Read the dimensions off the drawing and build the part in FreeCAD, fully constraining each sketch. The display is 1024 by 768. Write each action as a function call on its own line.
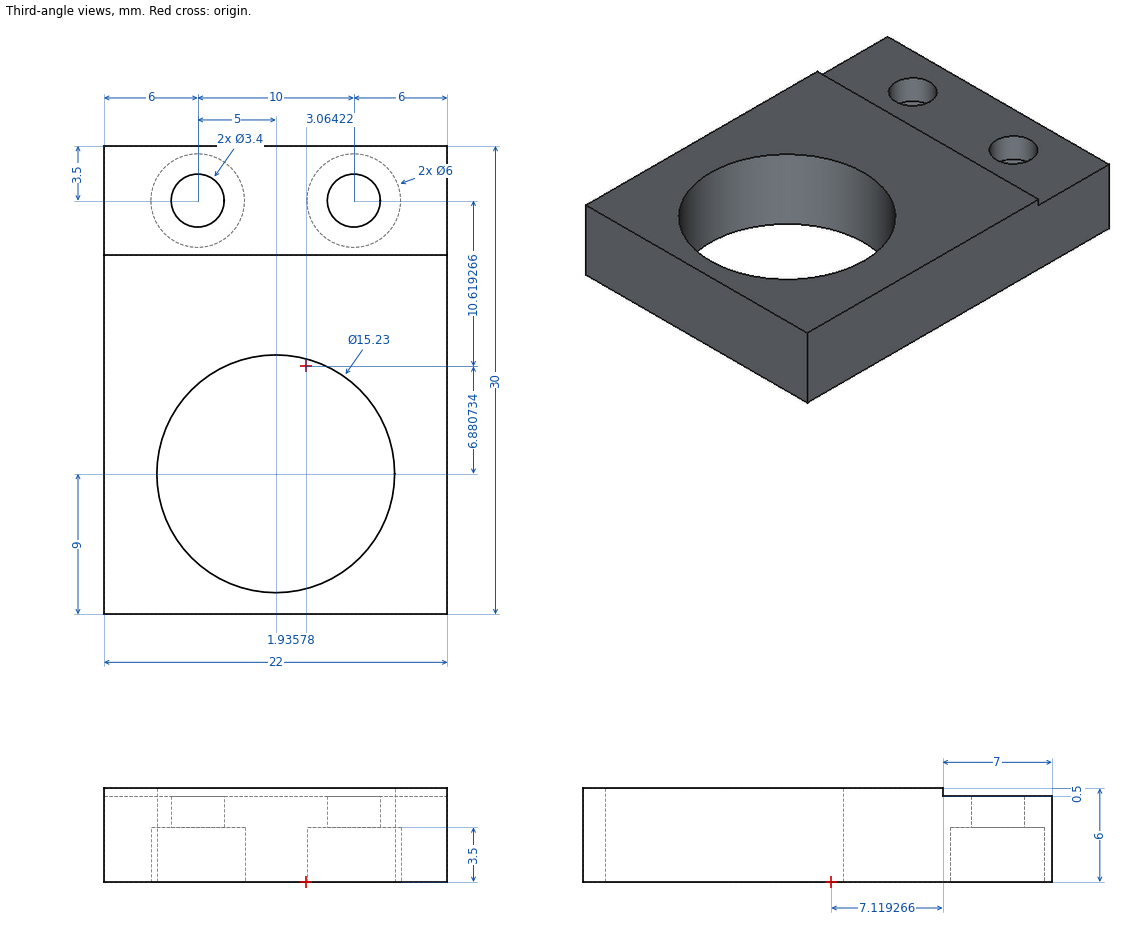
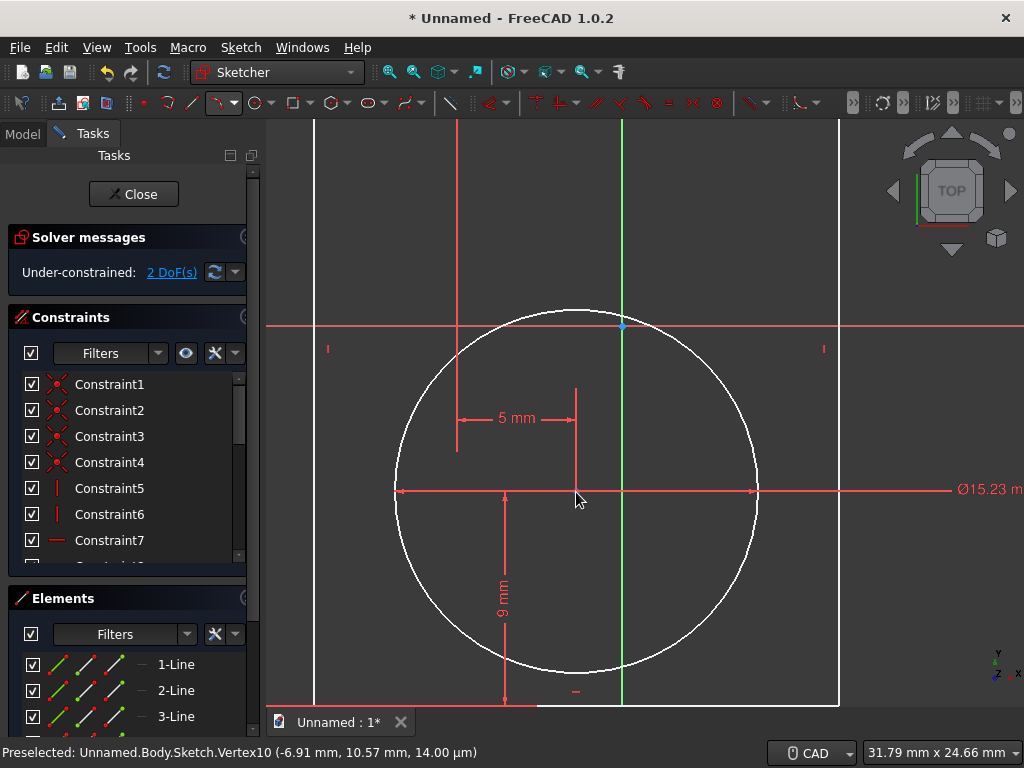
click(576, 491)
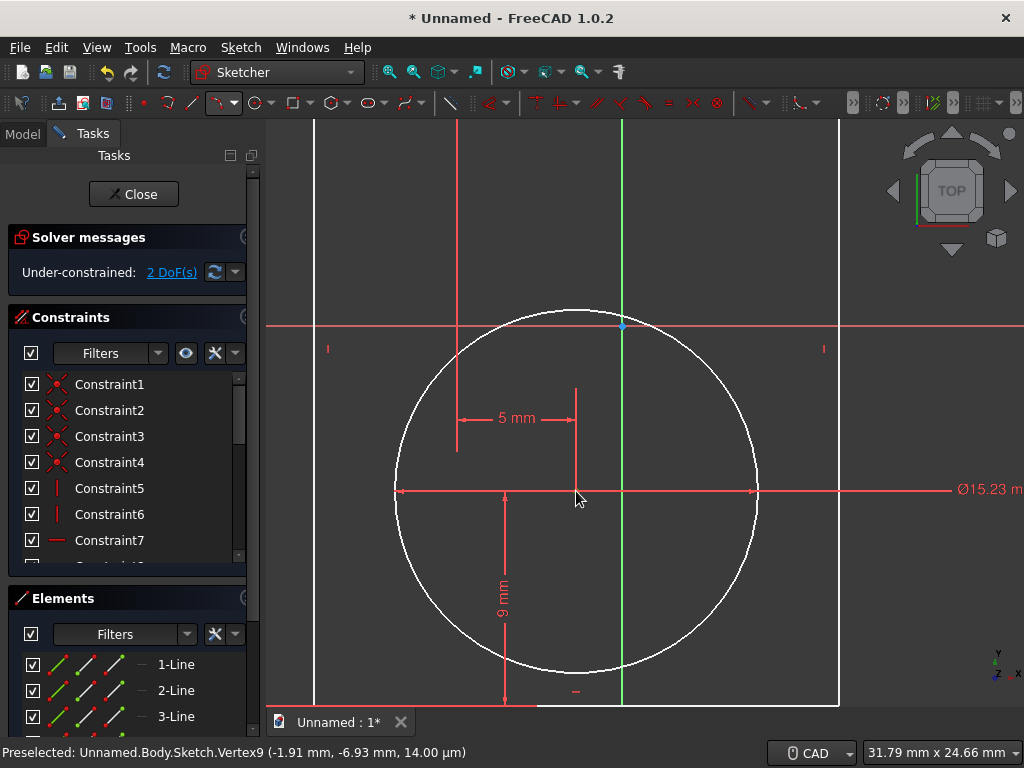
key(l)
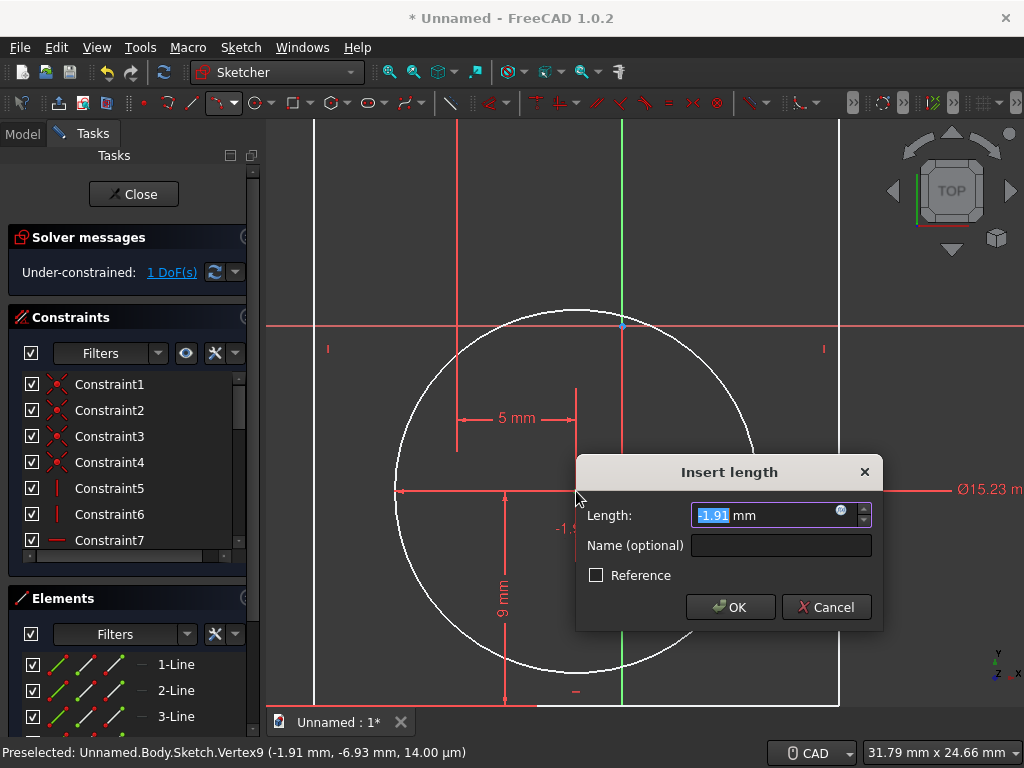
text(-1.93578)
key(Return)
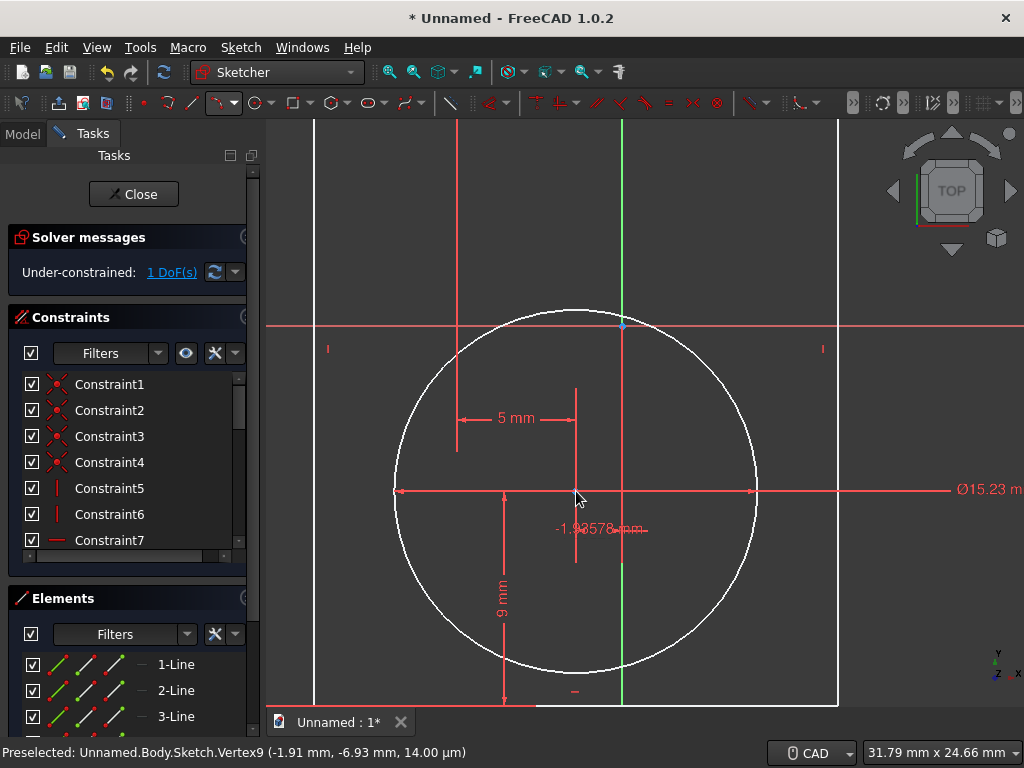
click(576, 491)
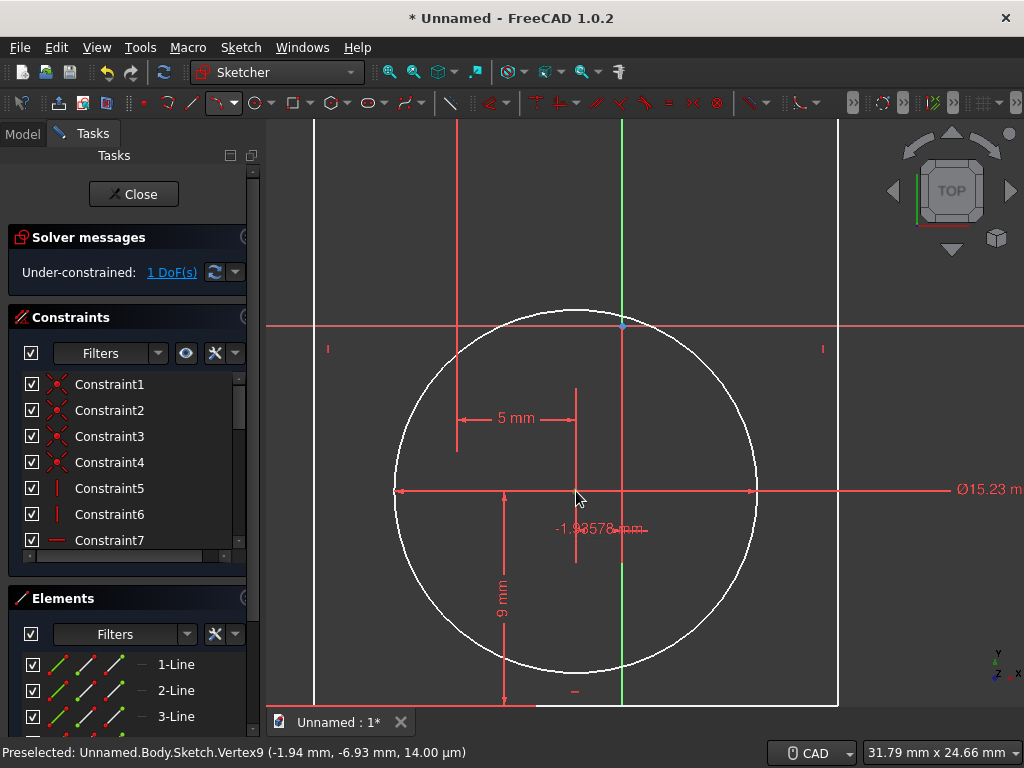
key(i)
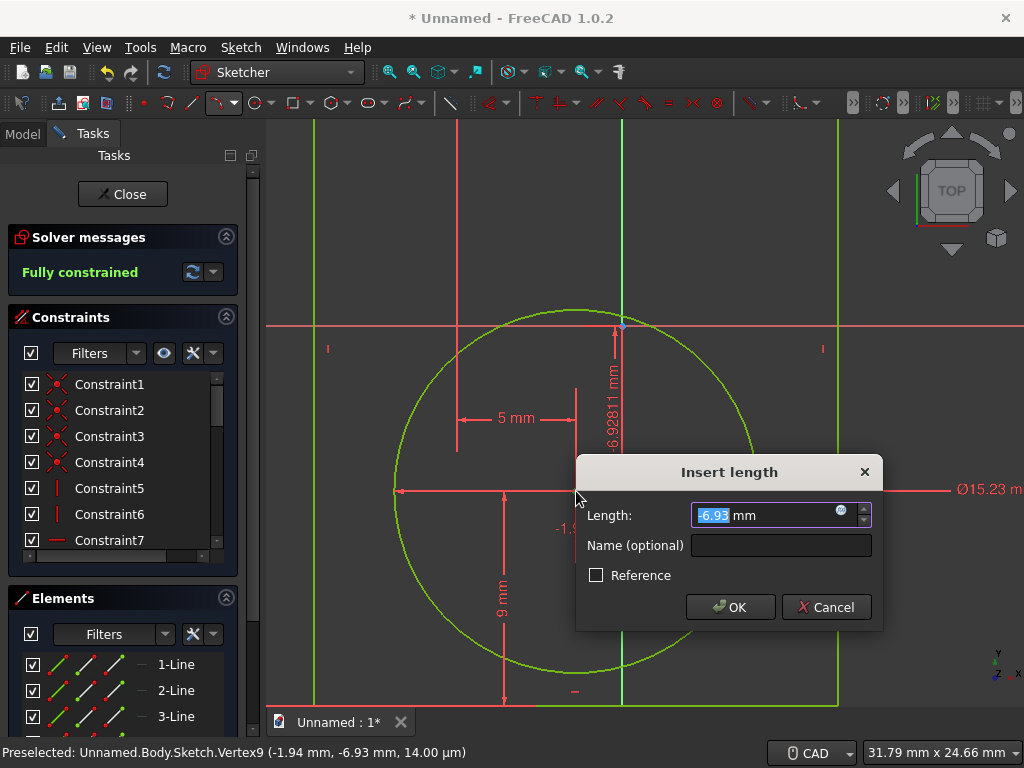
text(-6.880734)
key(Return)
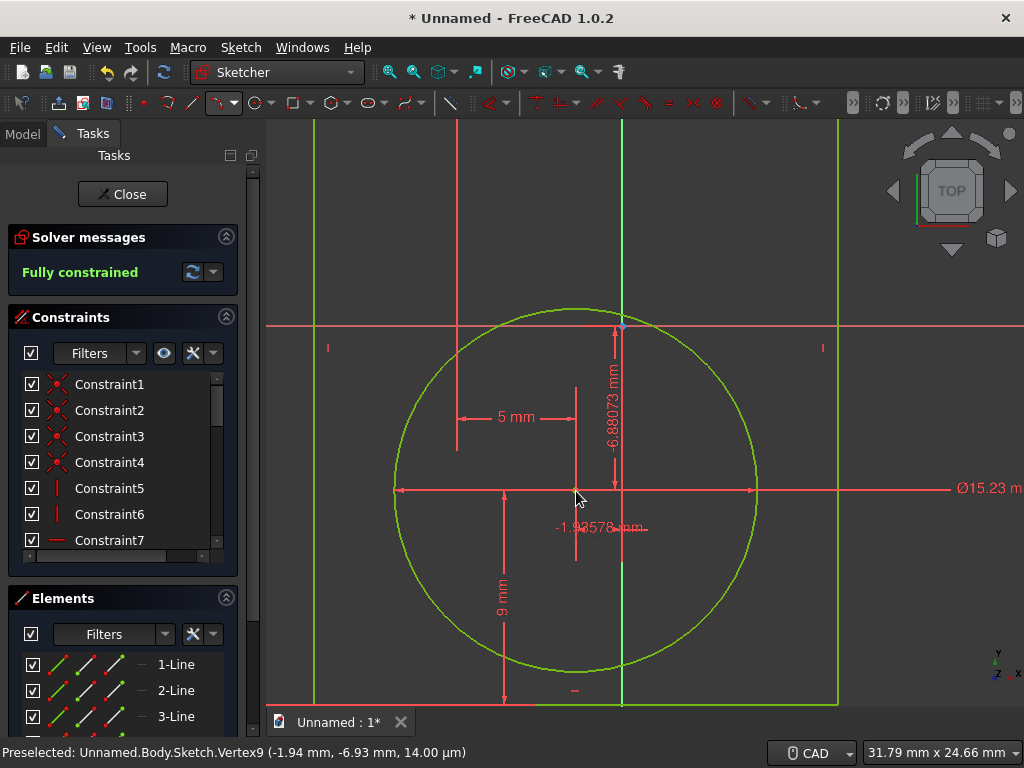
click(123, 194)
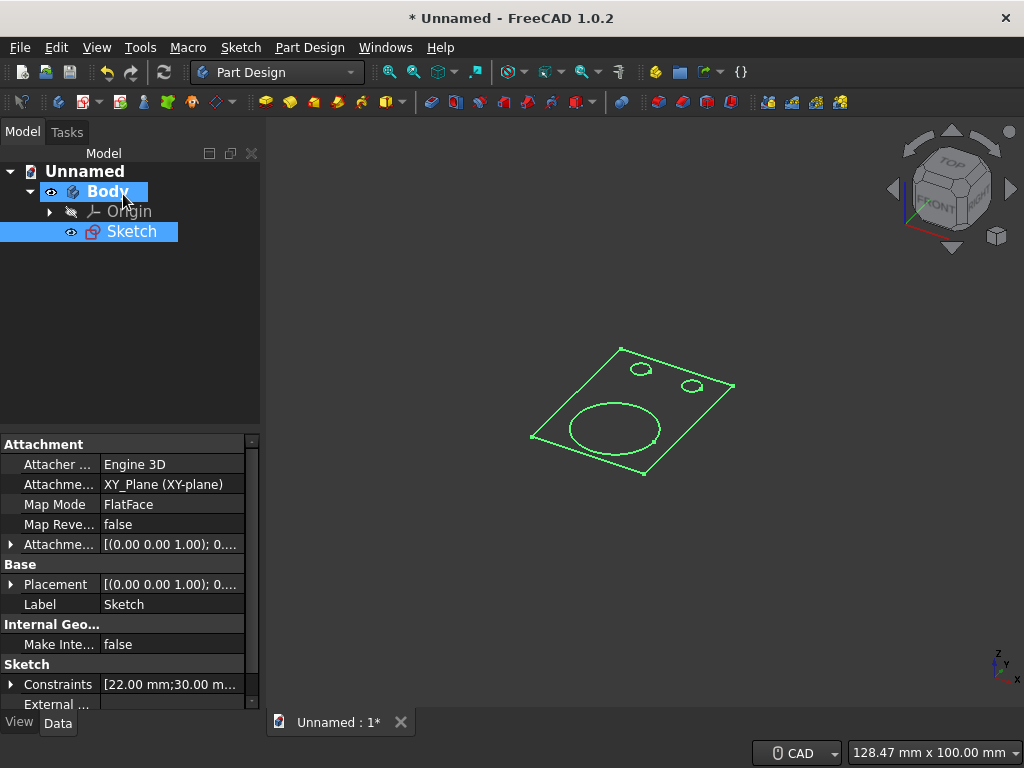
click(266, 102)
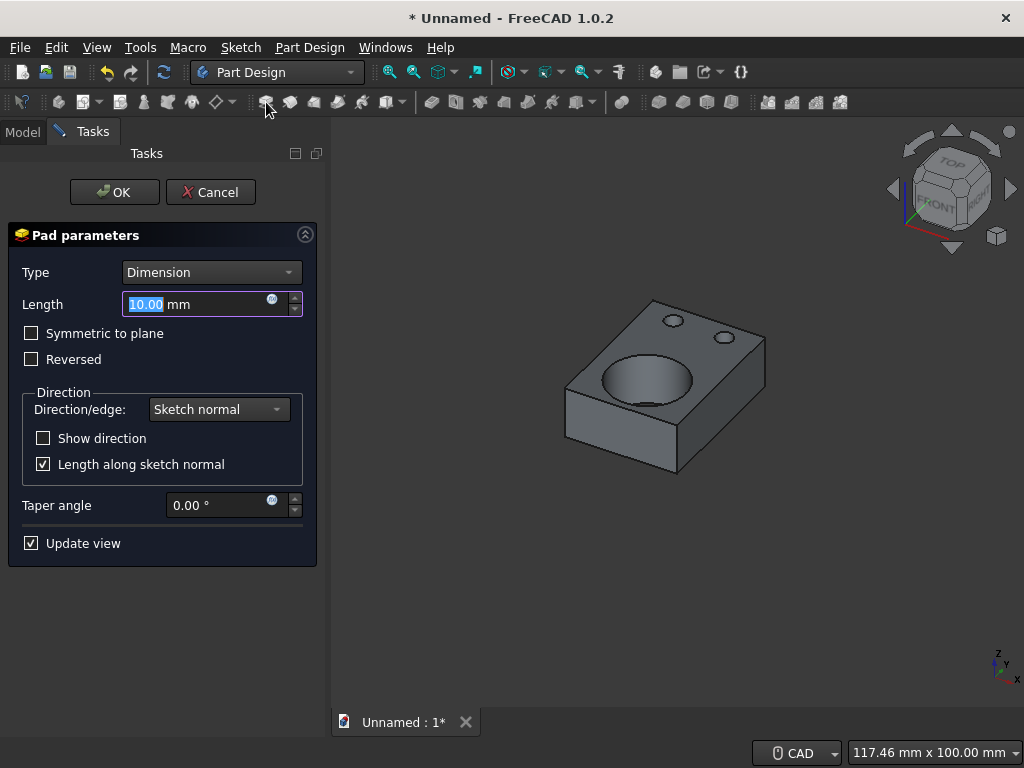
text(6)
key(Tab)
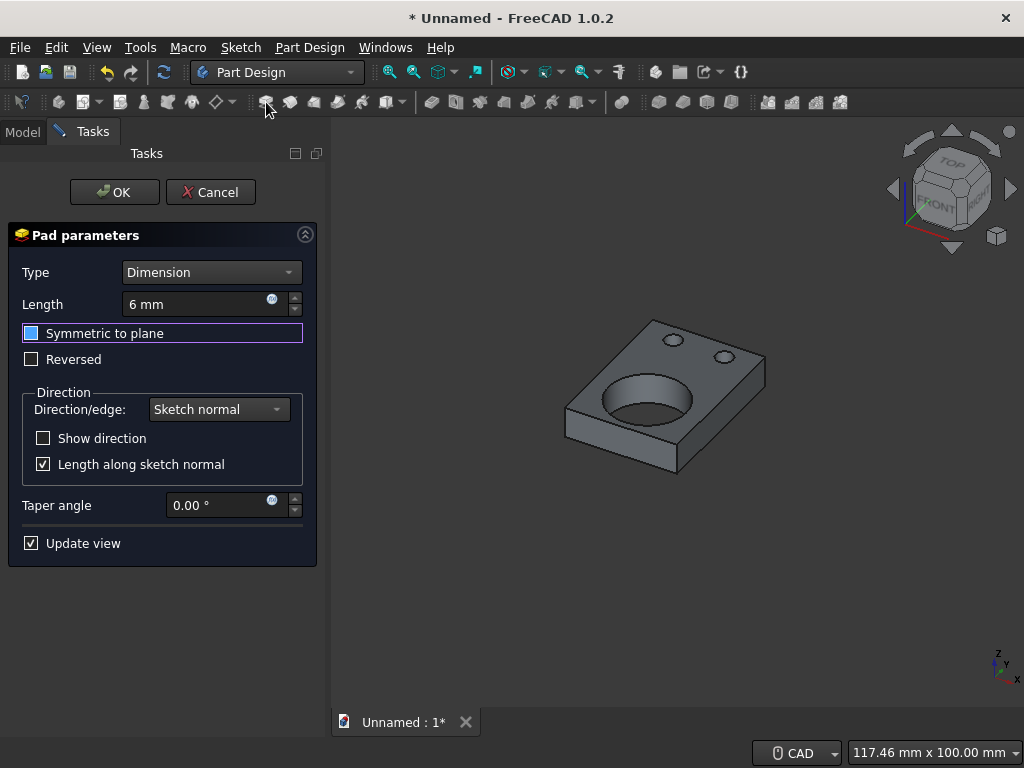
click(115, 192)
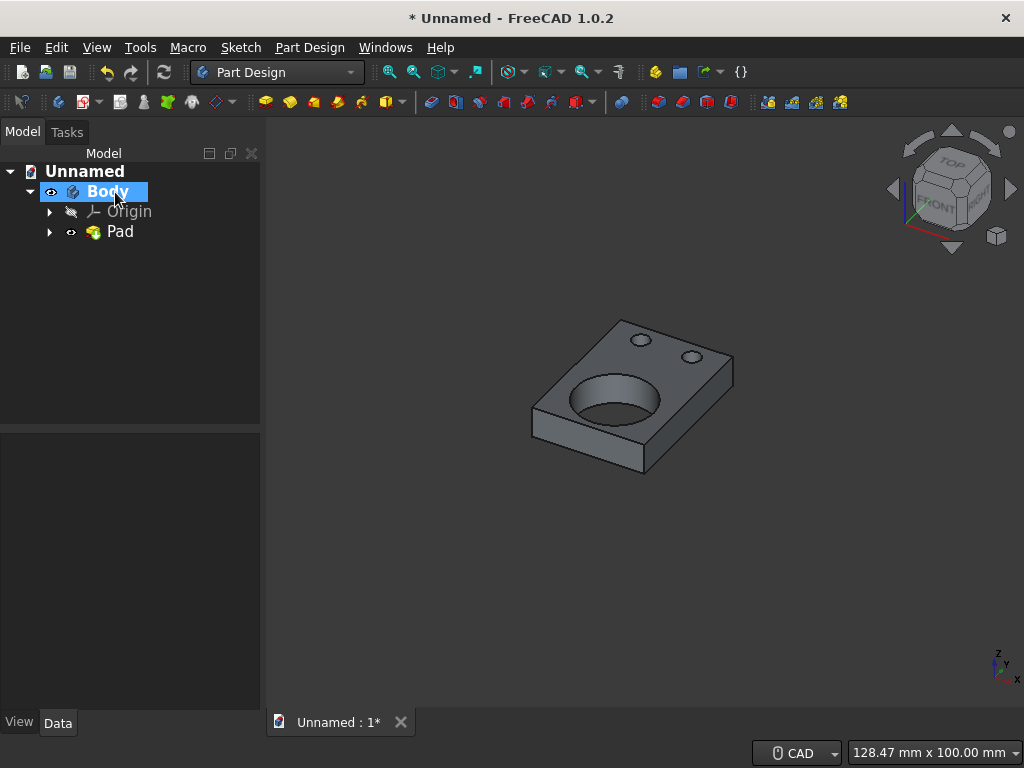
click(390, 72)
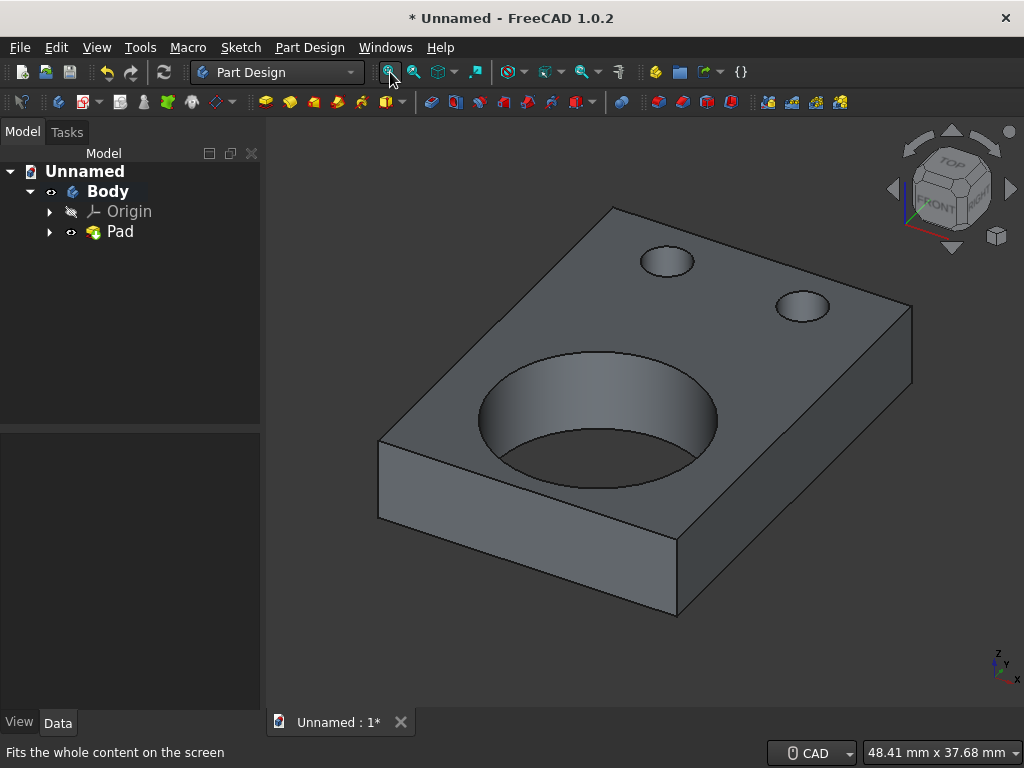
key(6)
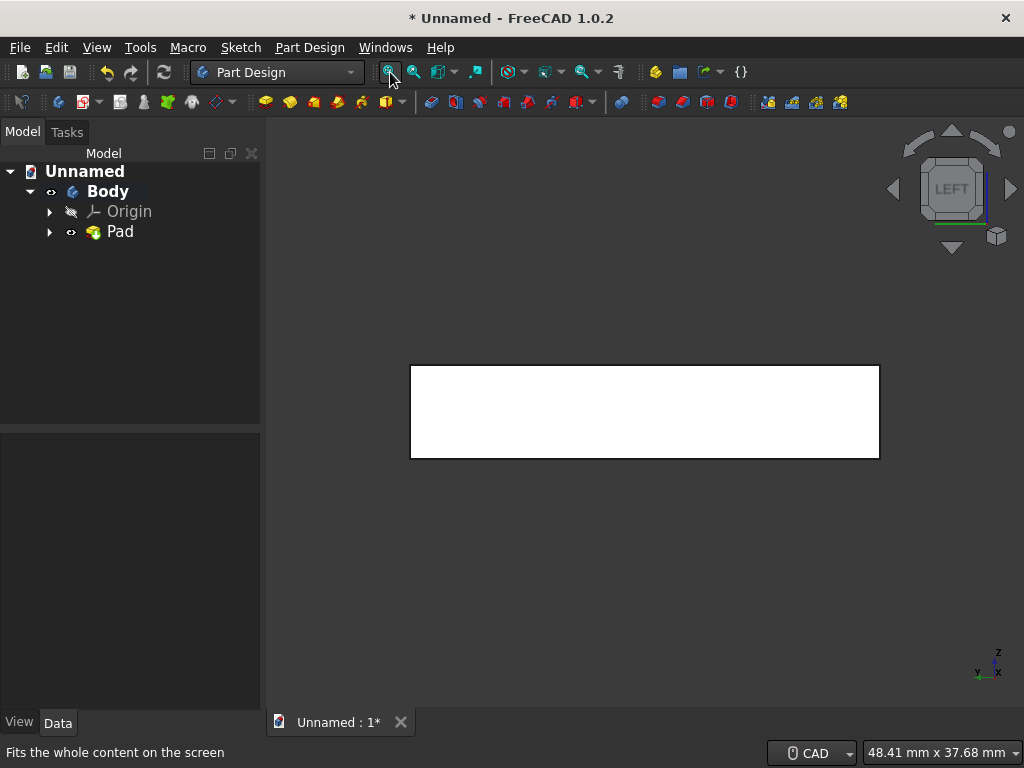
click(511, 411)